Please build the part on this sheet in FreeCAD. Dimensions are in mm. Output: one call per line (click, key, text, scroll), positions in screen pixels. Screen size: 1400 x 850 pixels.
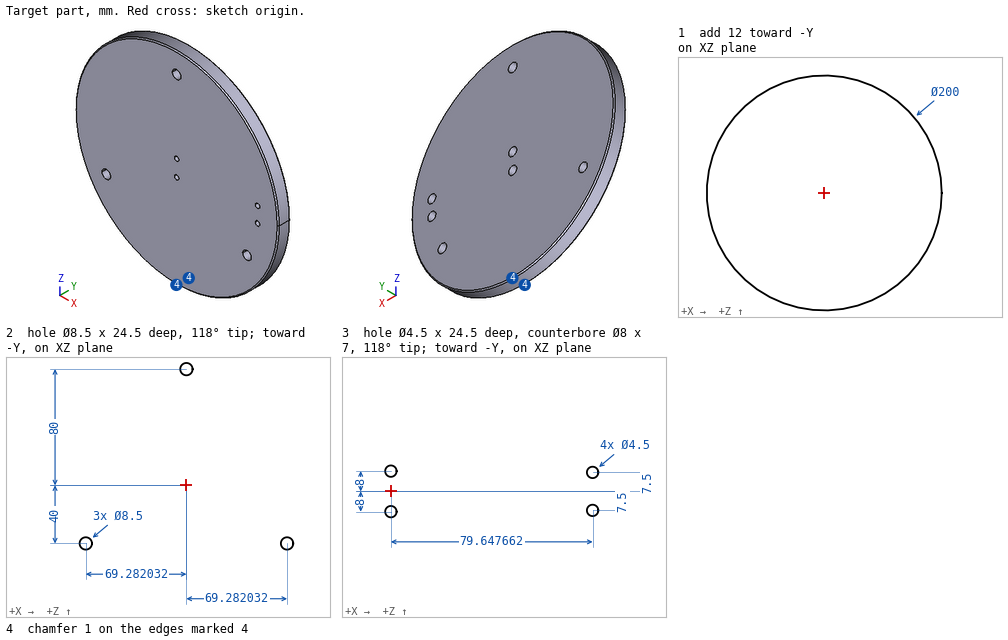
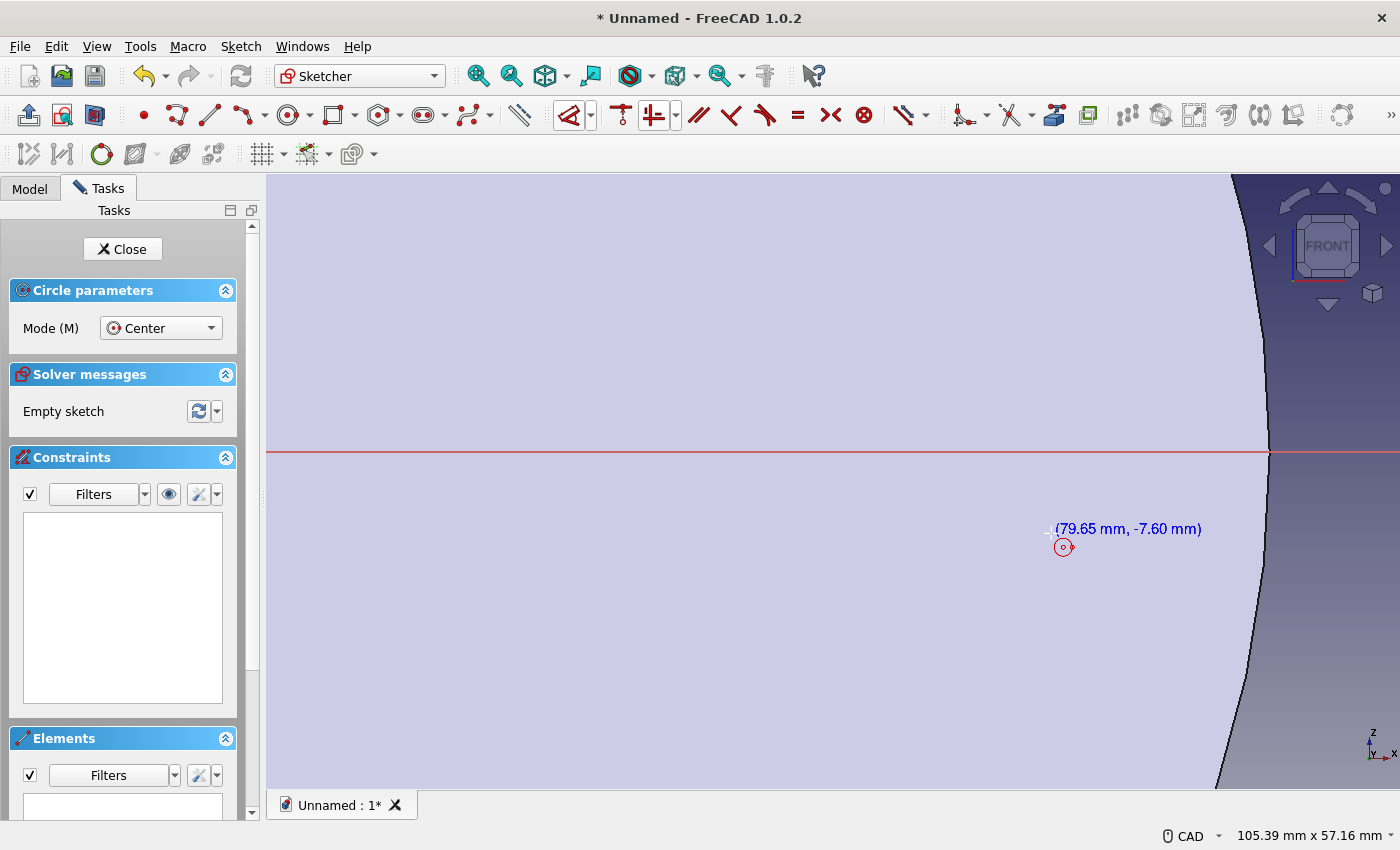
click(1051, 533)
move(1068, 516)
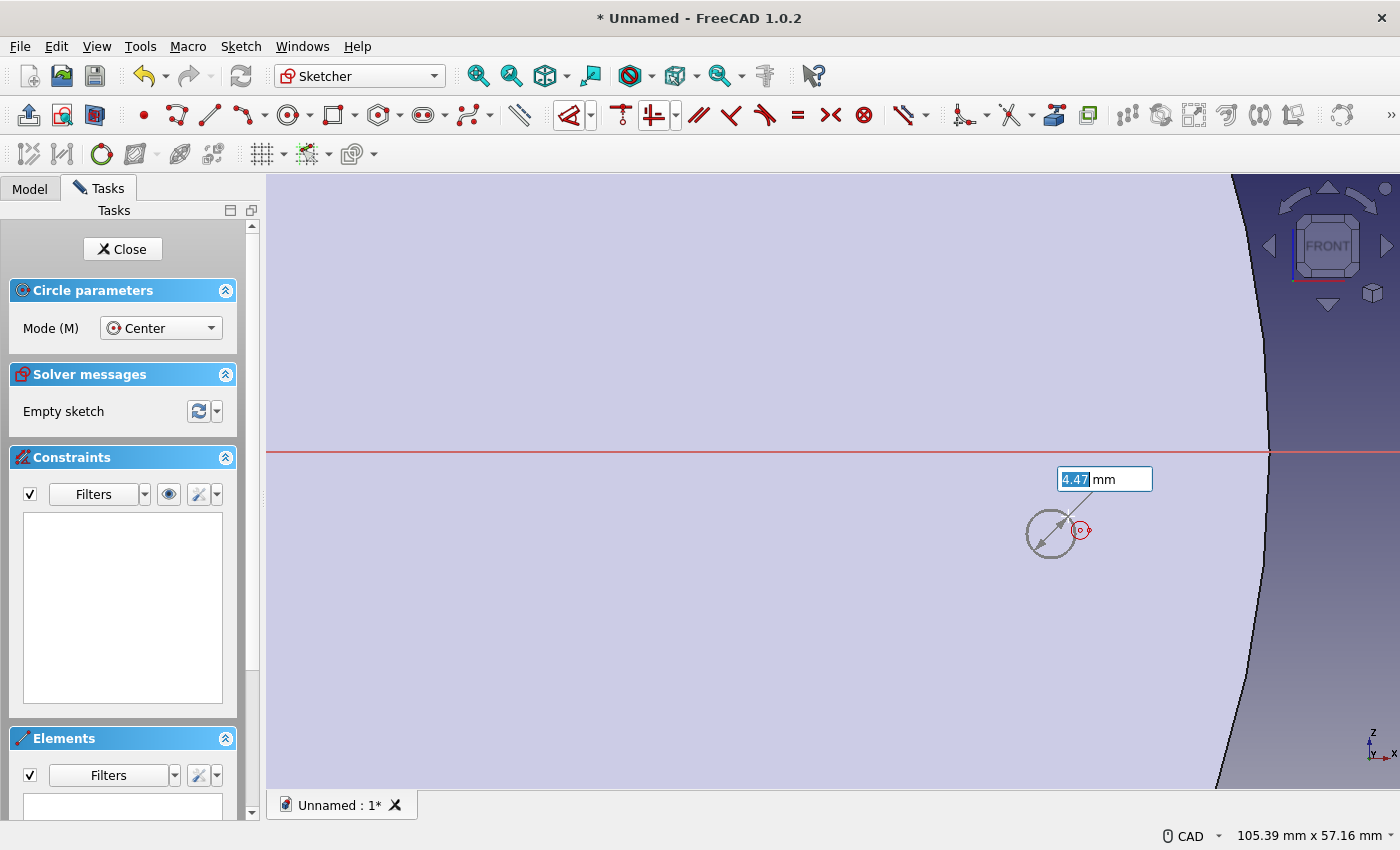
text(4.5)
key(Return)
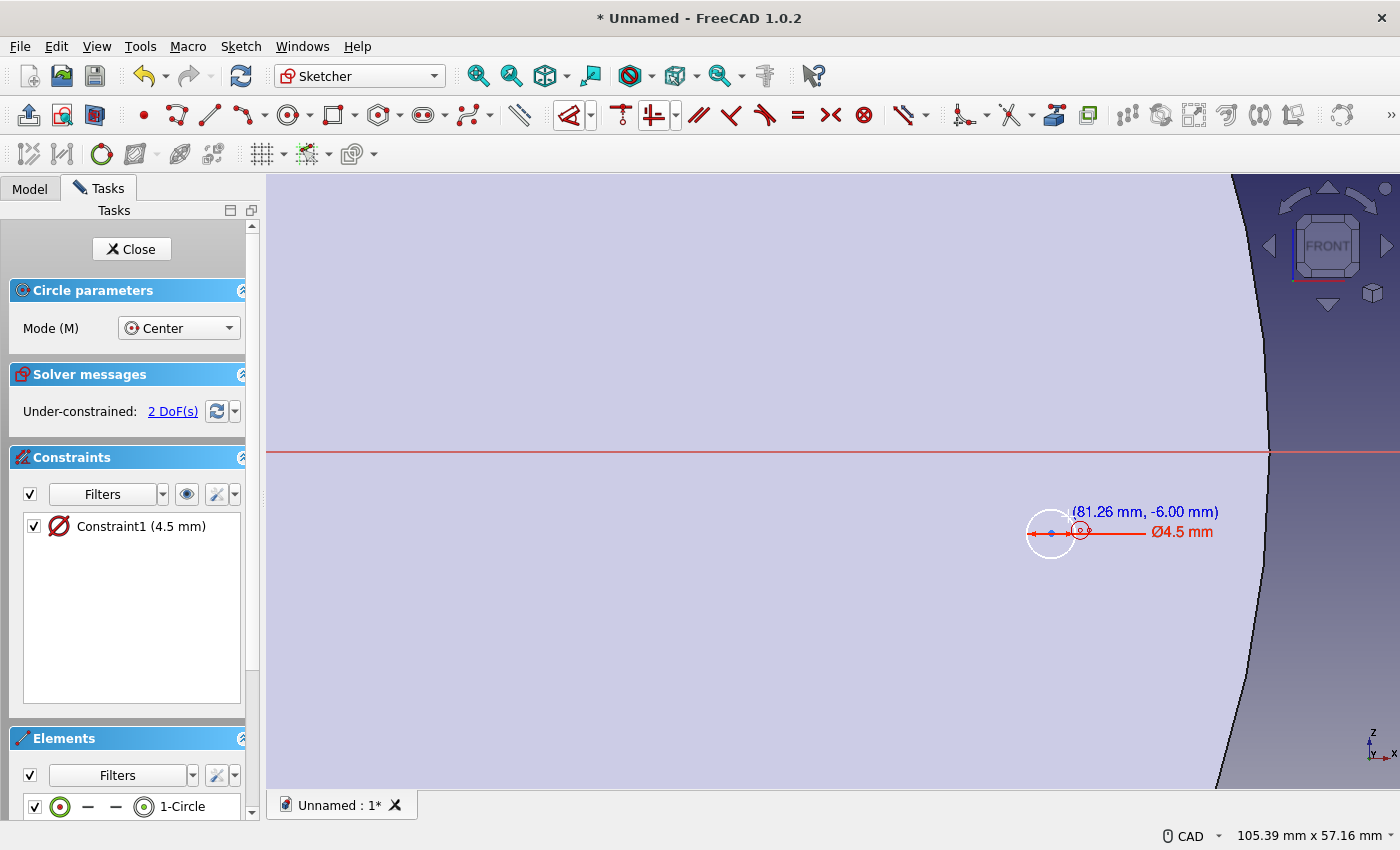
click(1051, 372)
move(1068, 355)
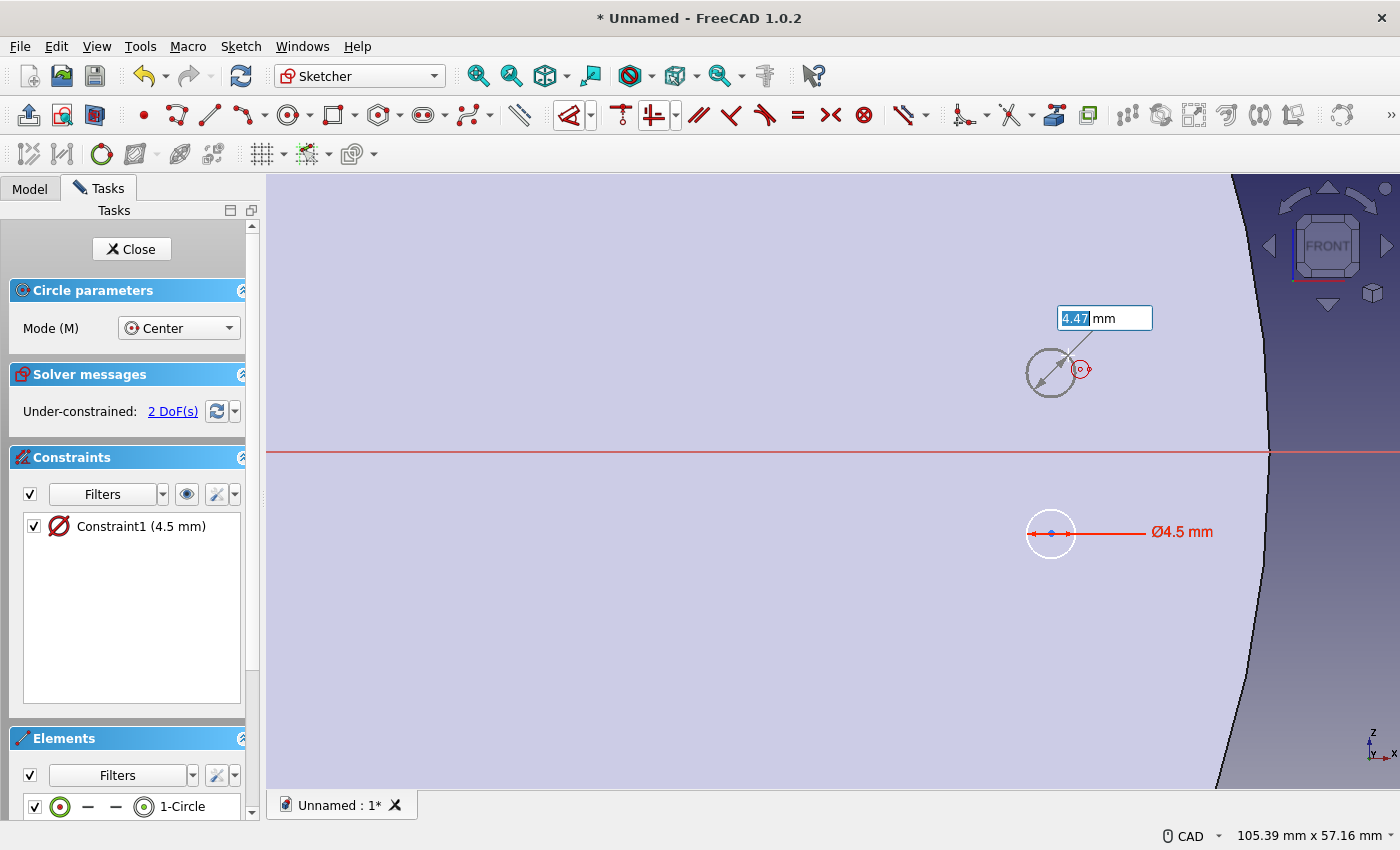
text(4.5)
key(Return)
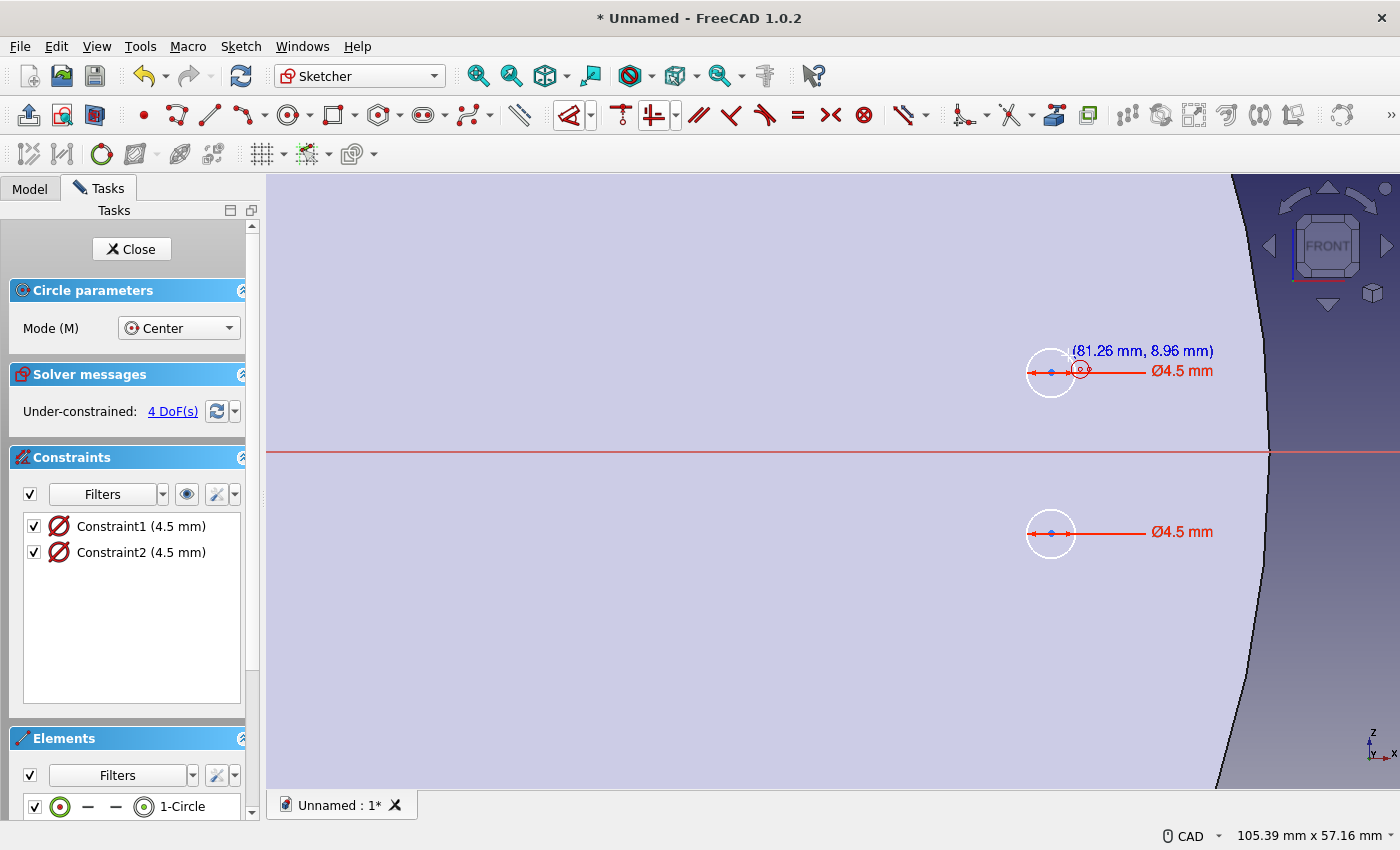
scroll(1054, 541, down, 2)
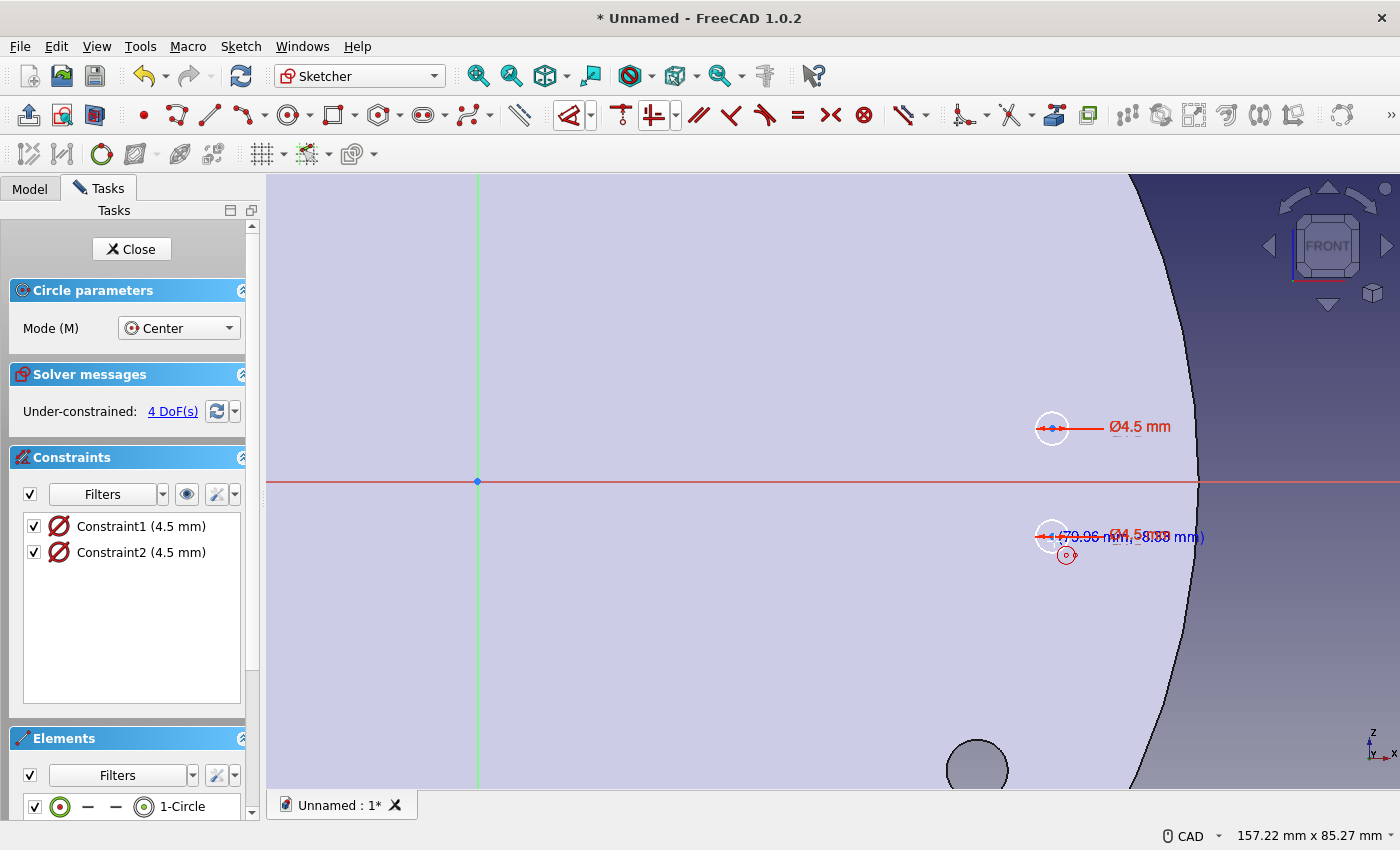
scroll(478, 424, up, 2)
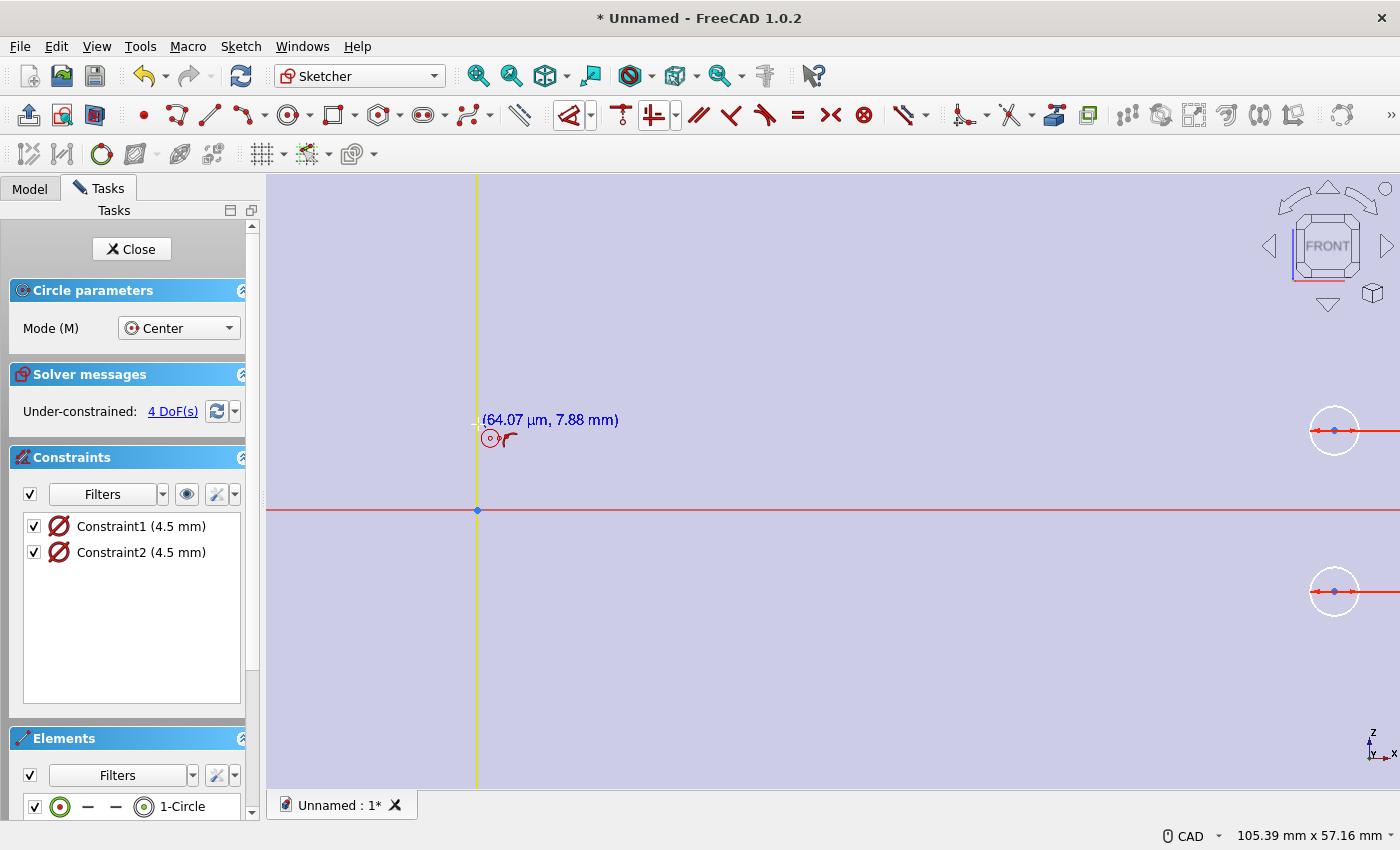
click(477, 424)
move(494, 407)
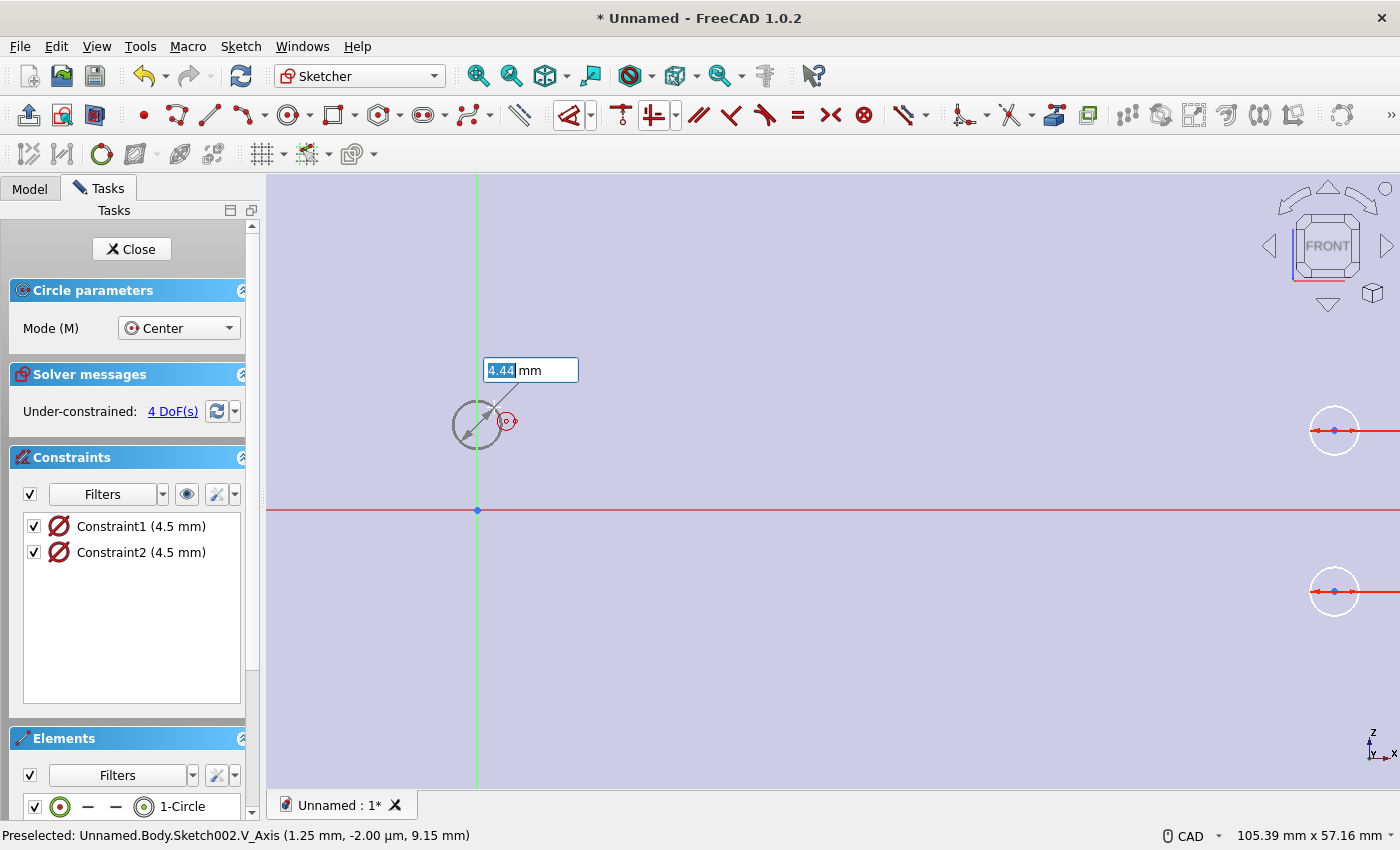
text(4.5)
key(Return)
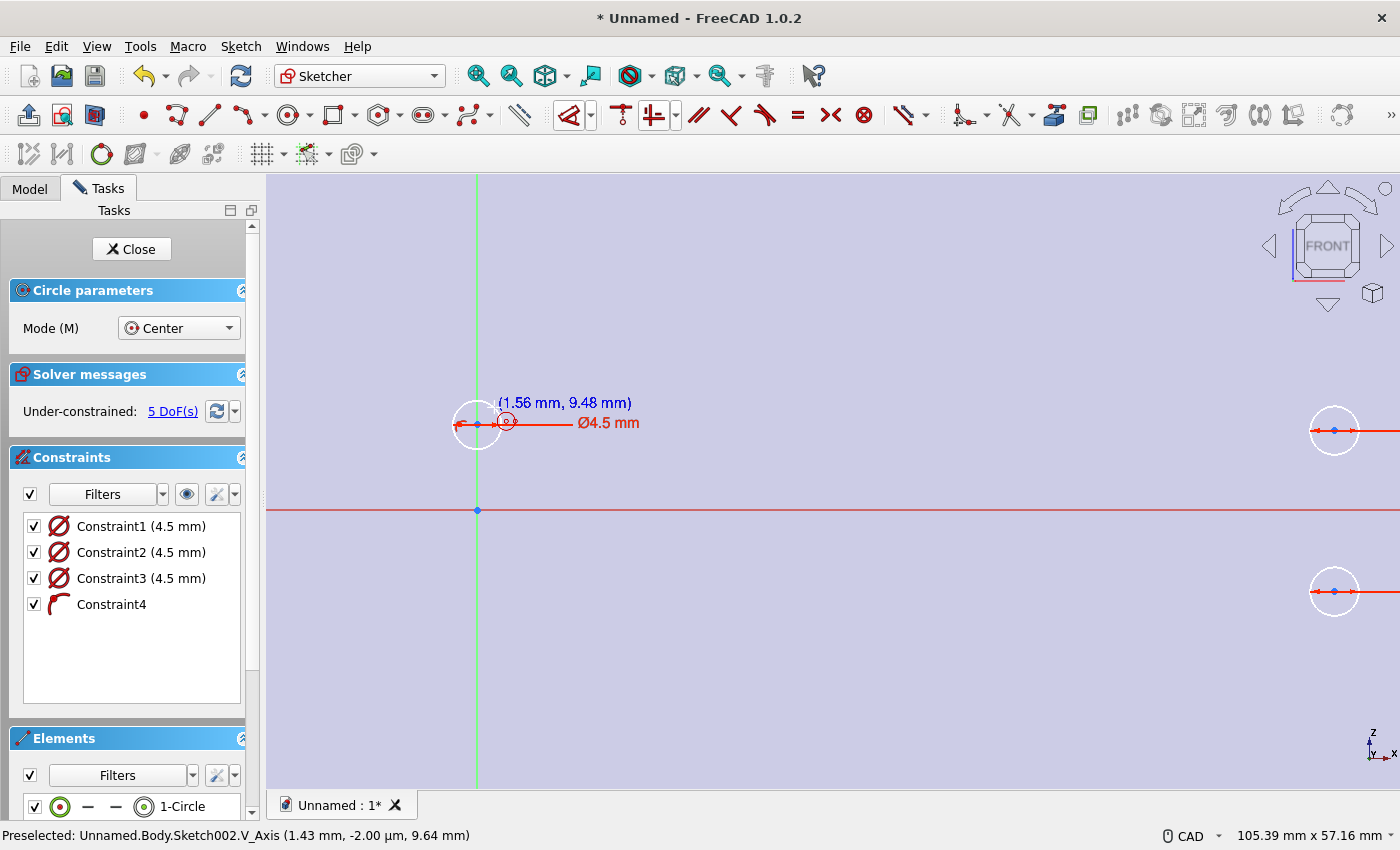
click(477, 596)
move(494, 579)